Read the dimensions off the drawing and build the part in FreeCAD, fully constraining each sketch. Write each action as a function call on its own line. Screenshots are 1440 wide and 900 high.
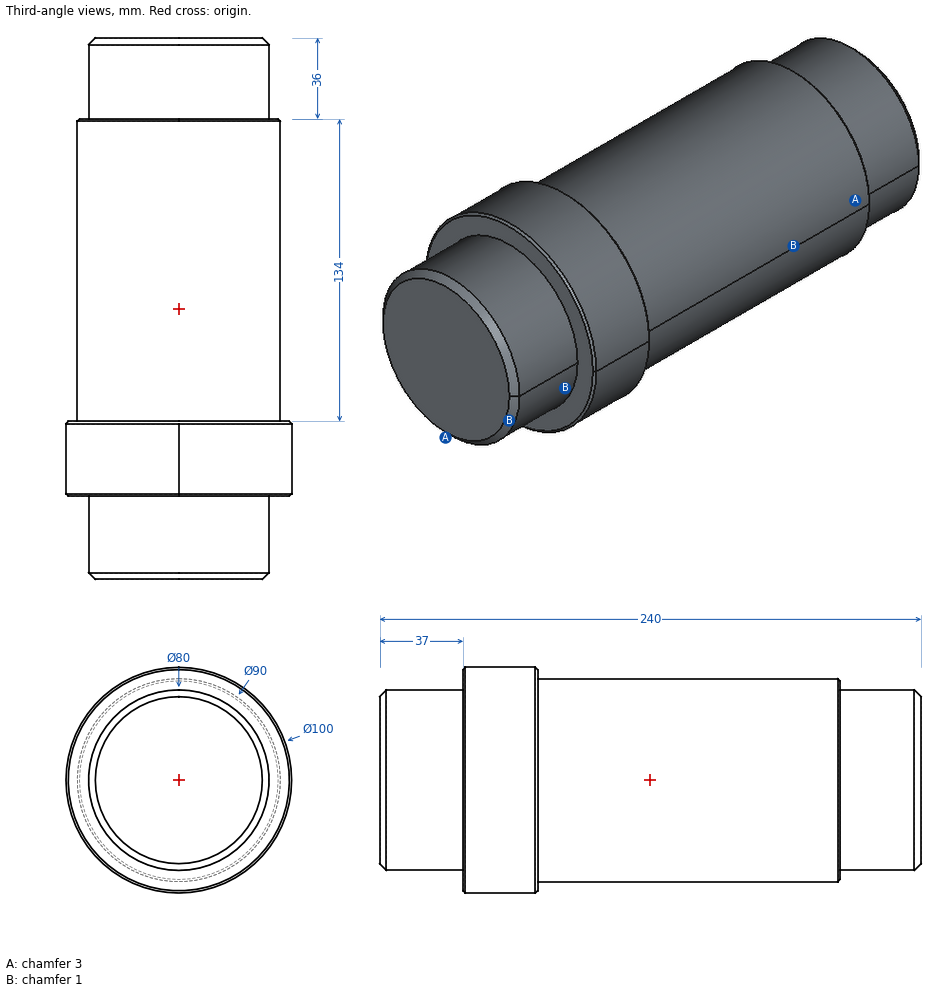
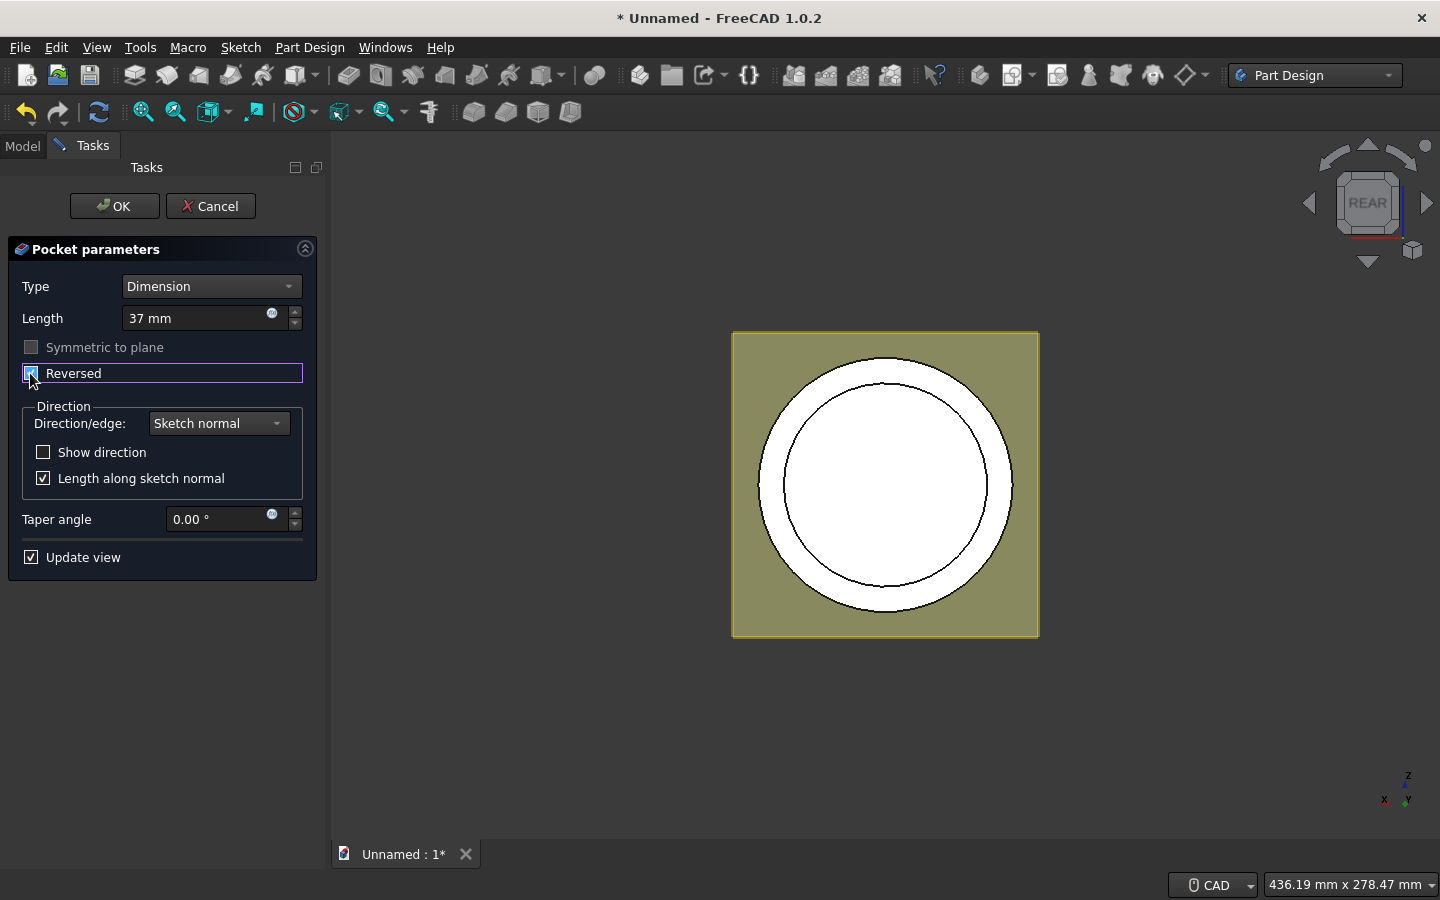
click(115, 206)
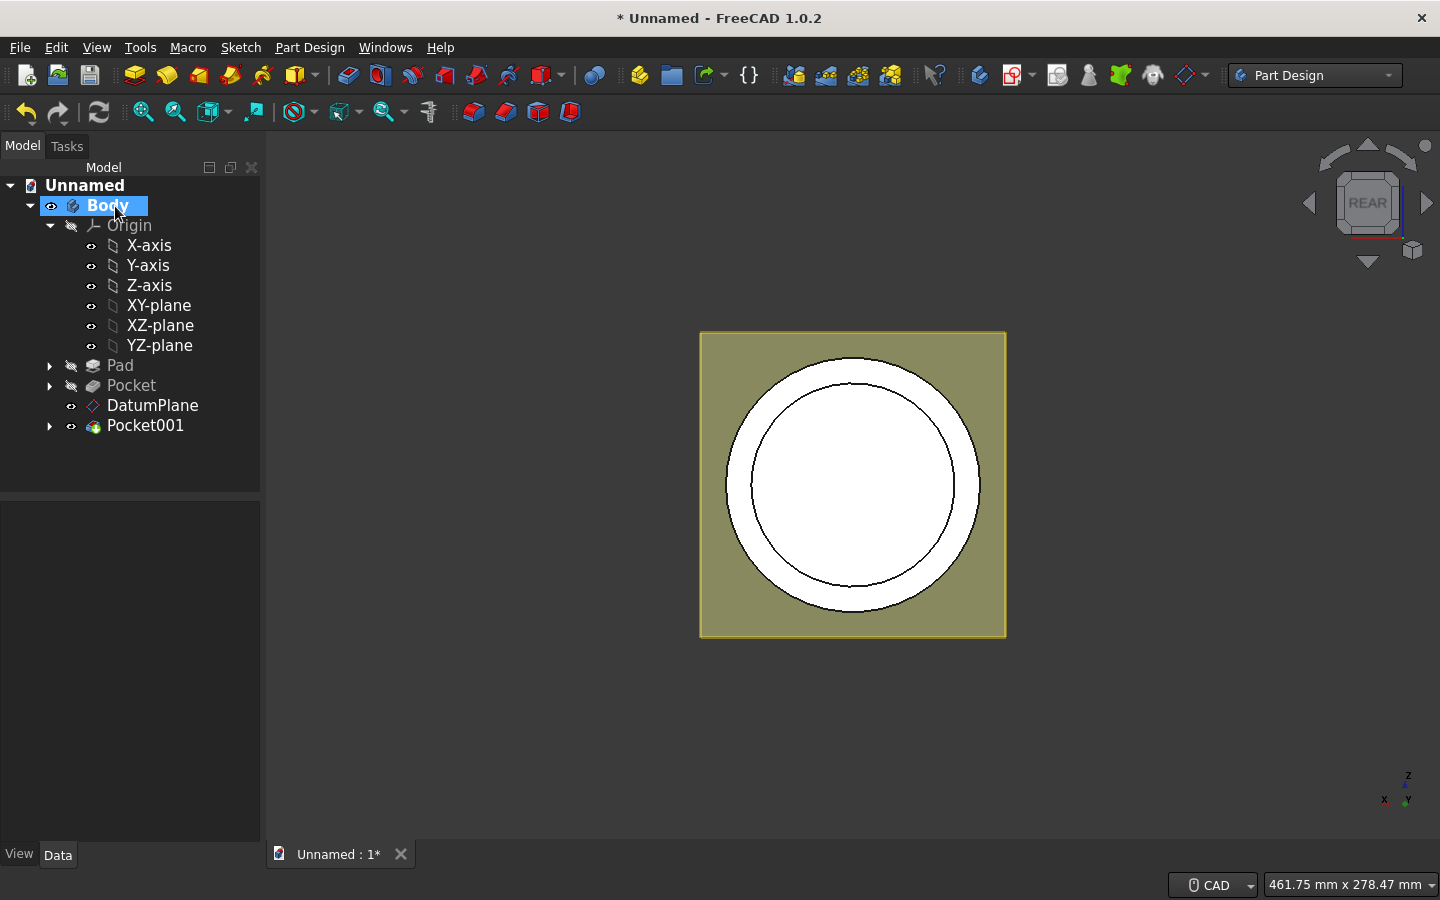
click(116, 406)
key(space)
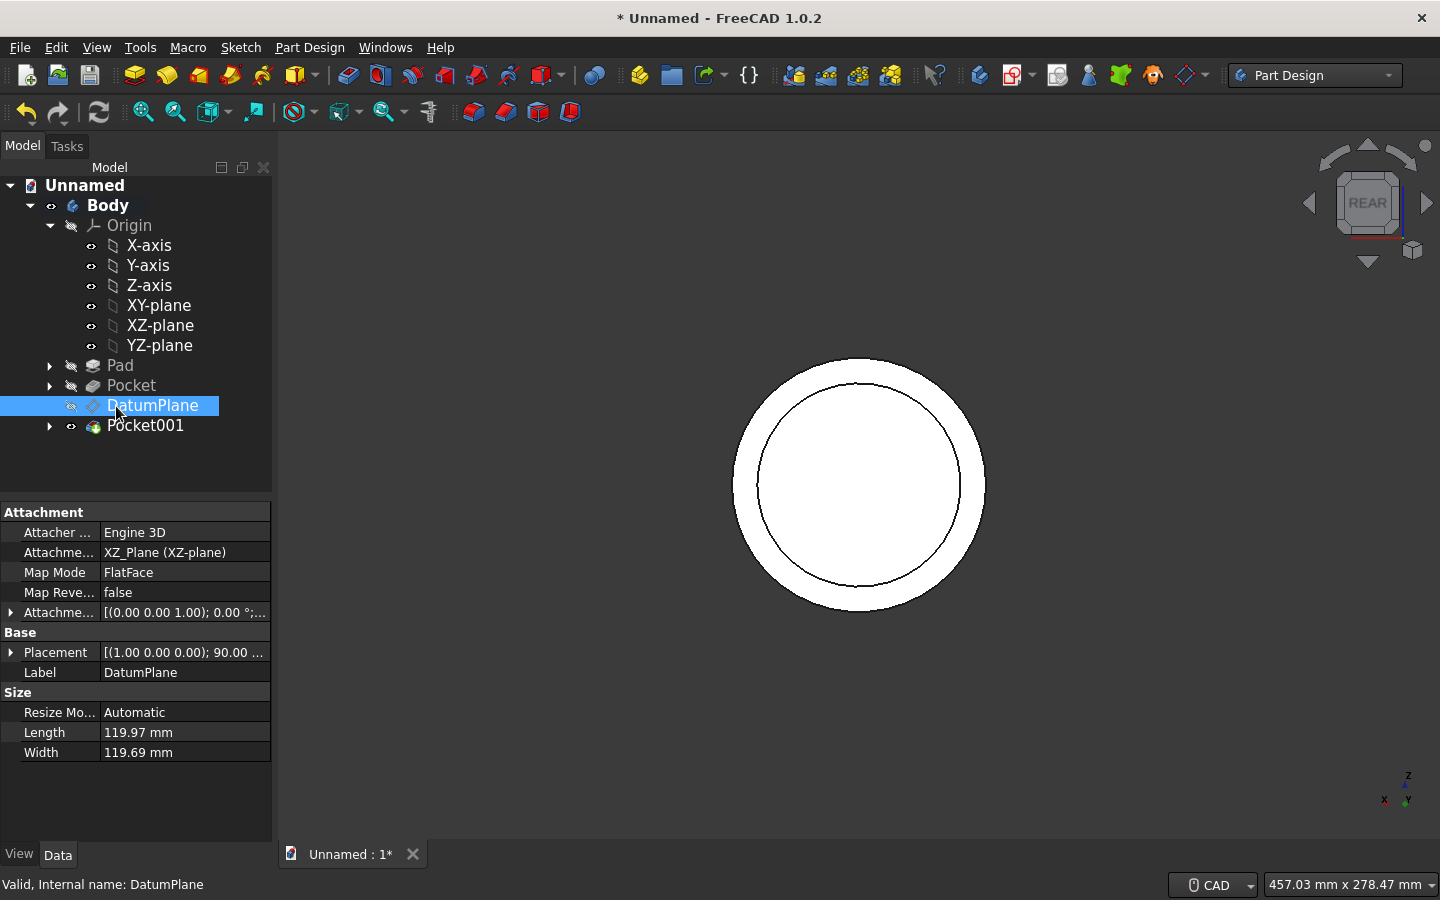
click(144, 112)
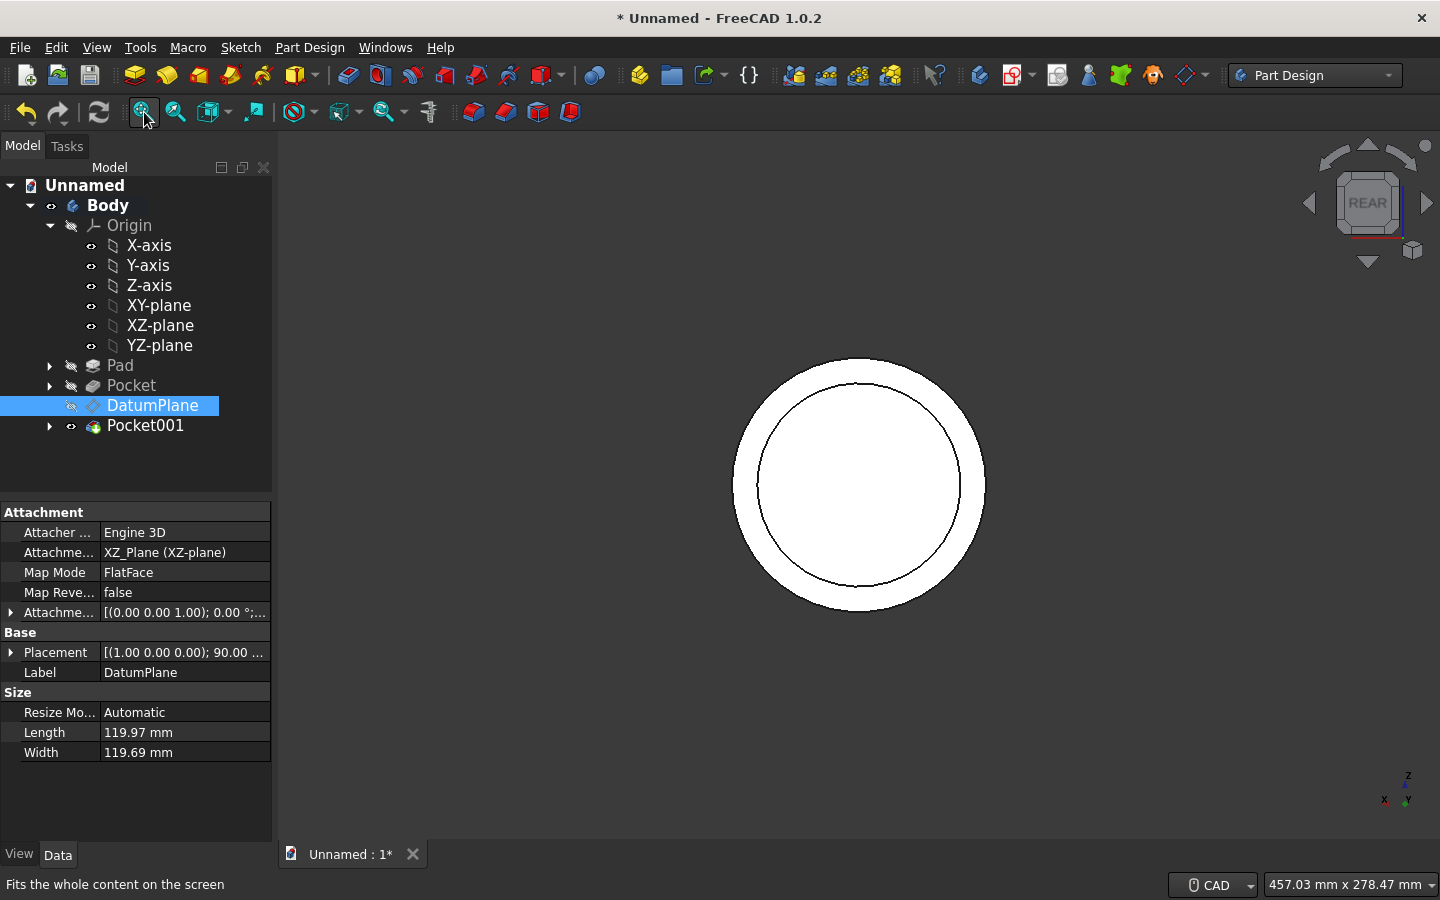
click(823, 593)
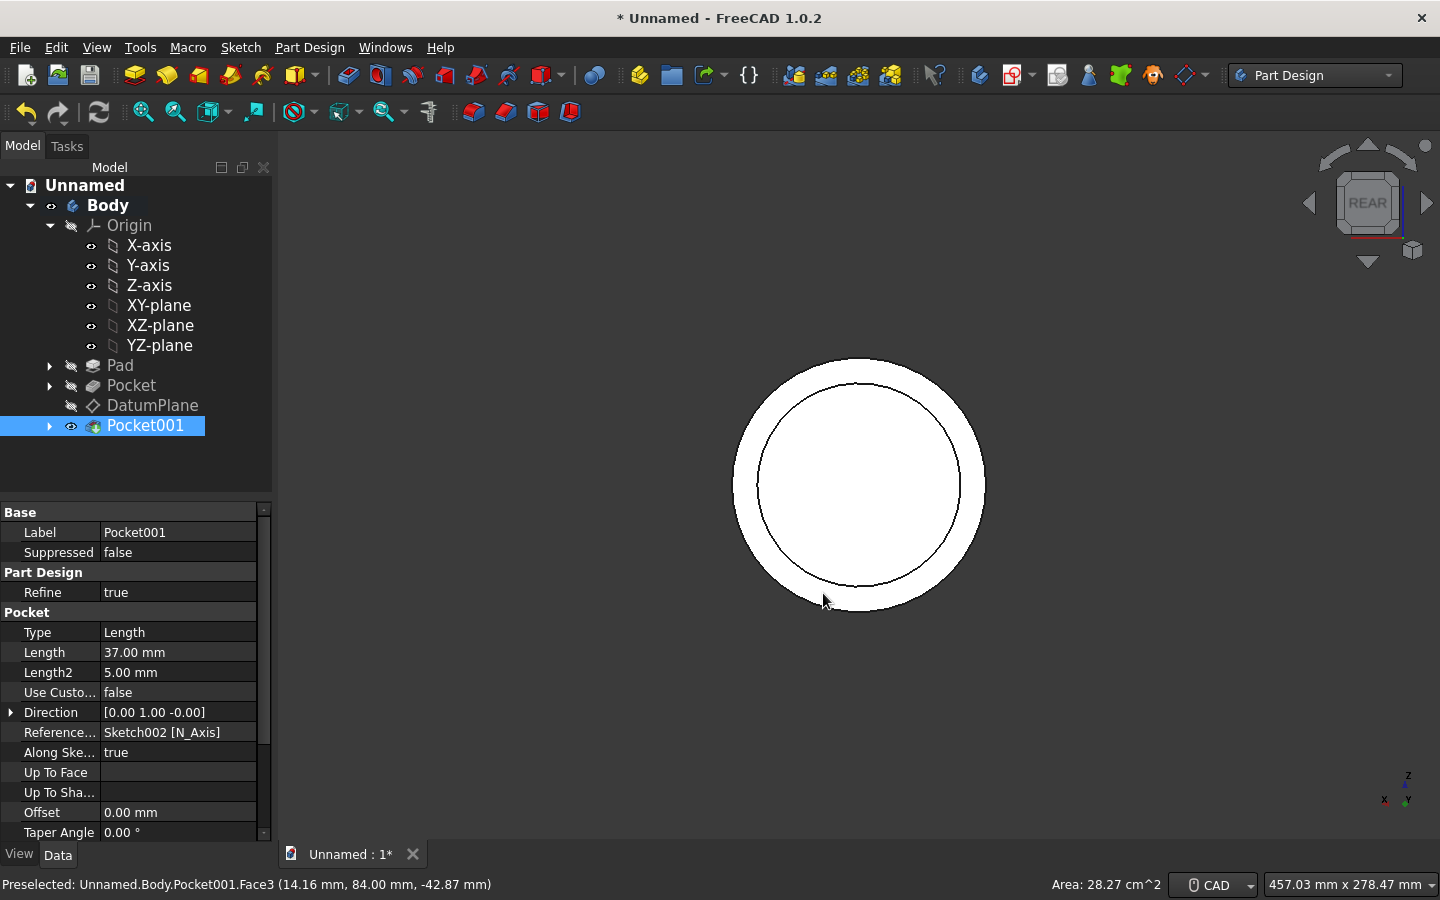
click(1012, 76)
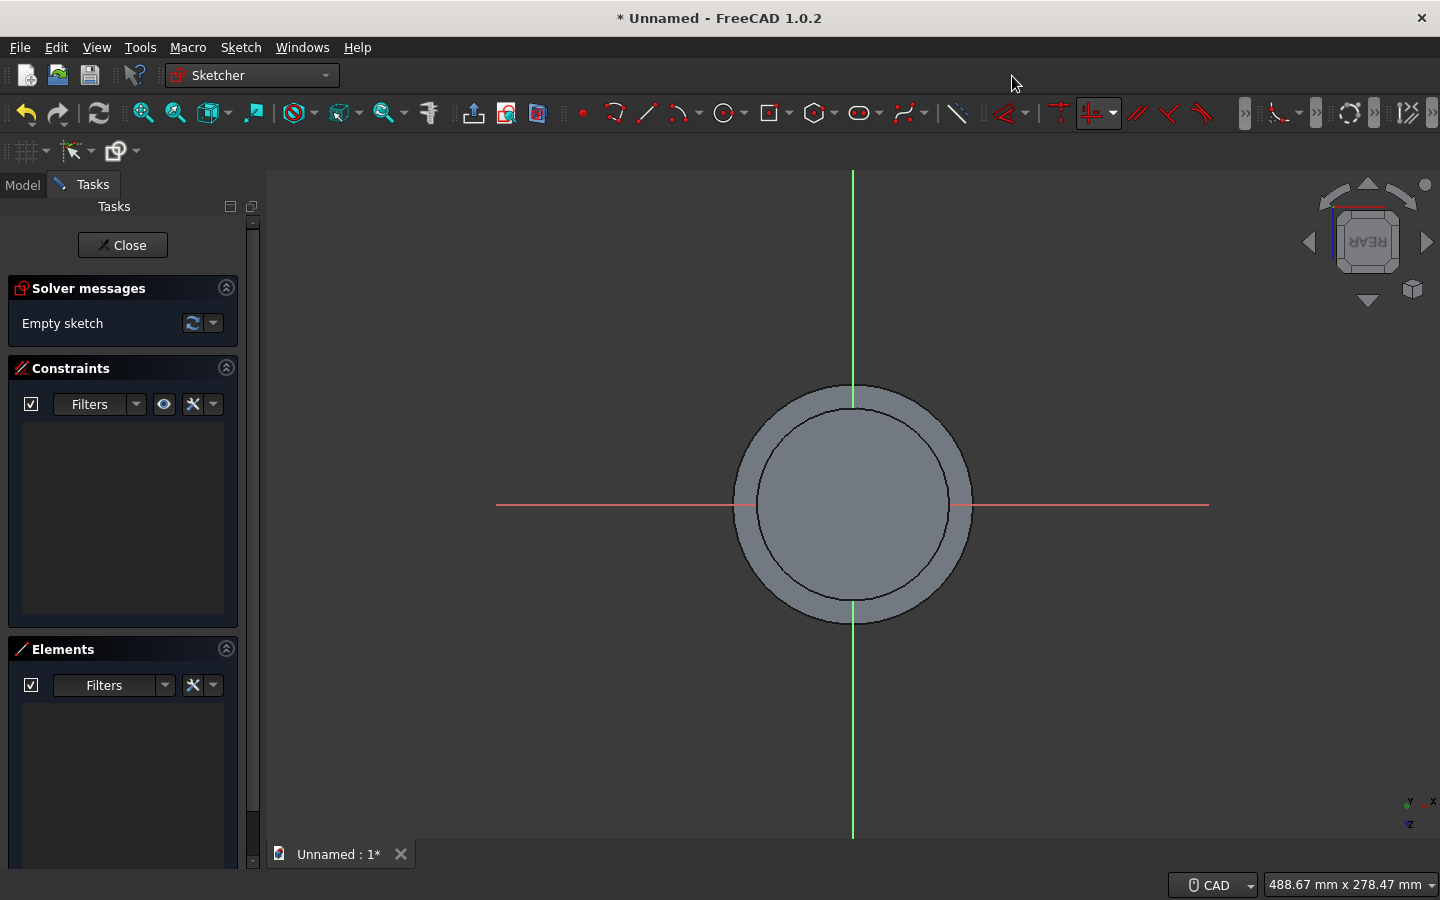
click(538, 114)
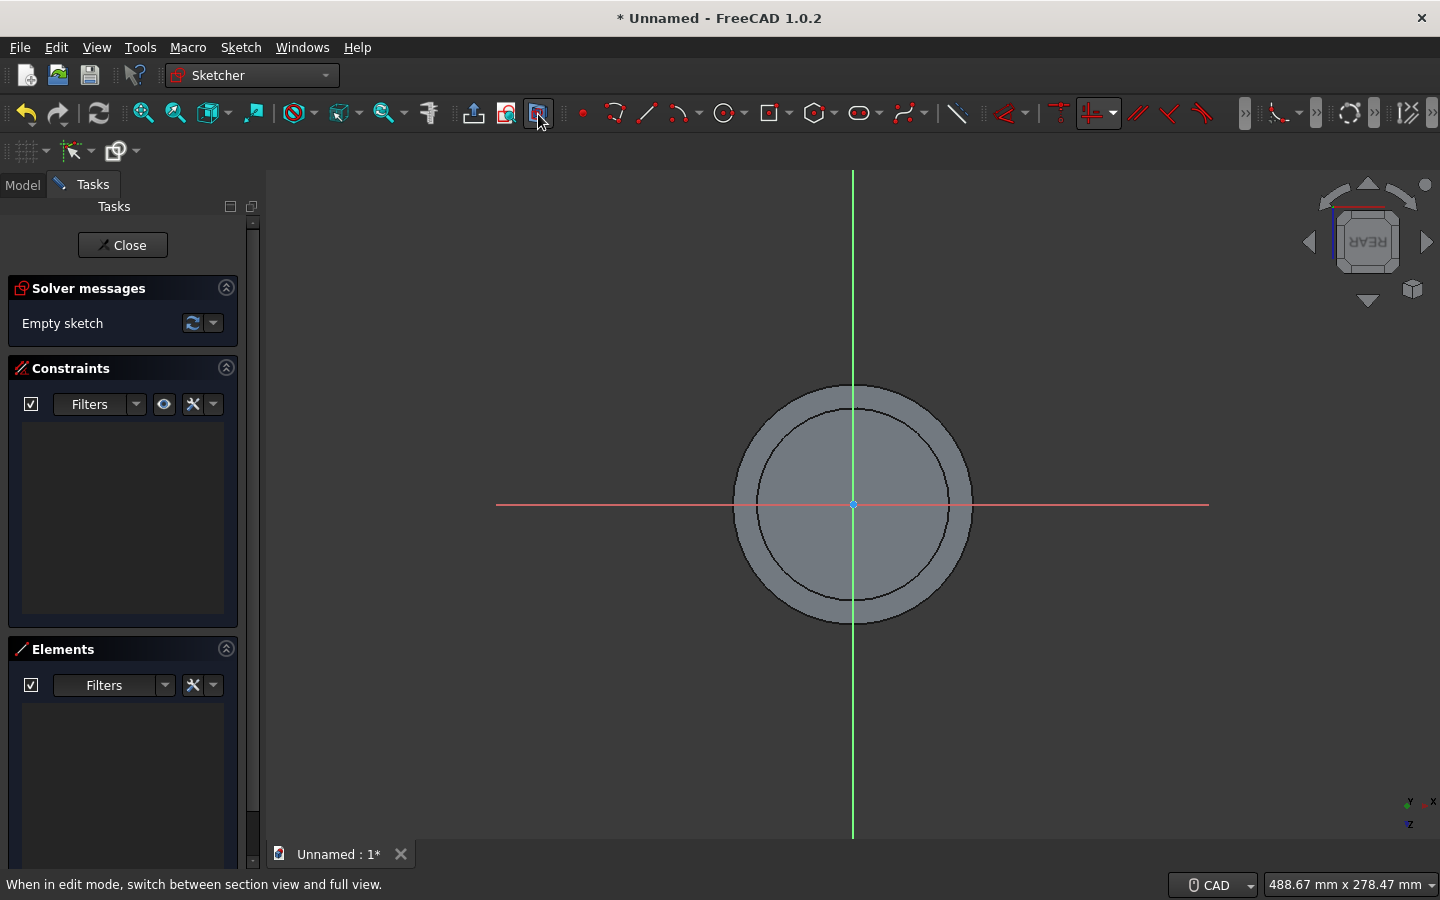
scroll(936, 505, up, 3)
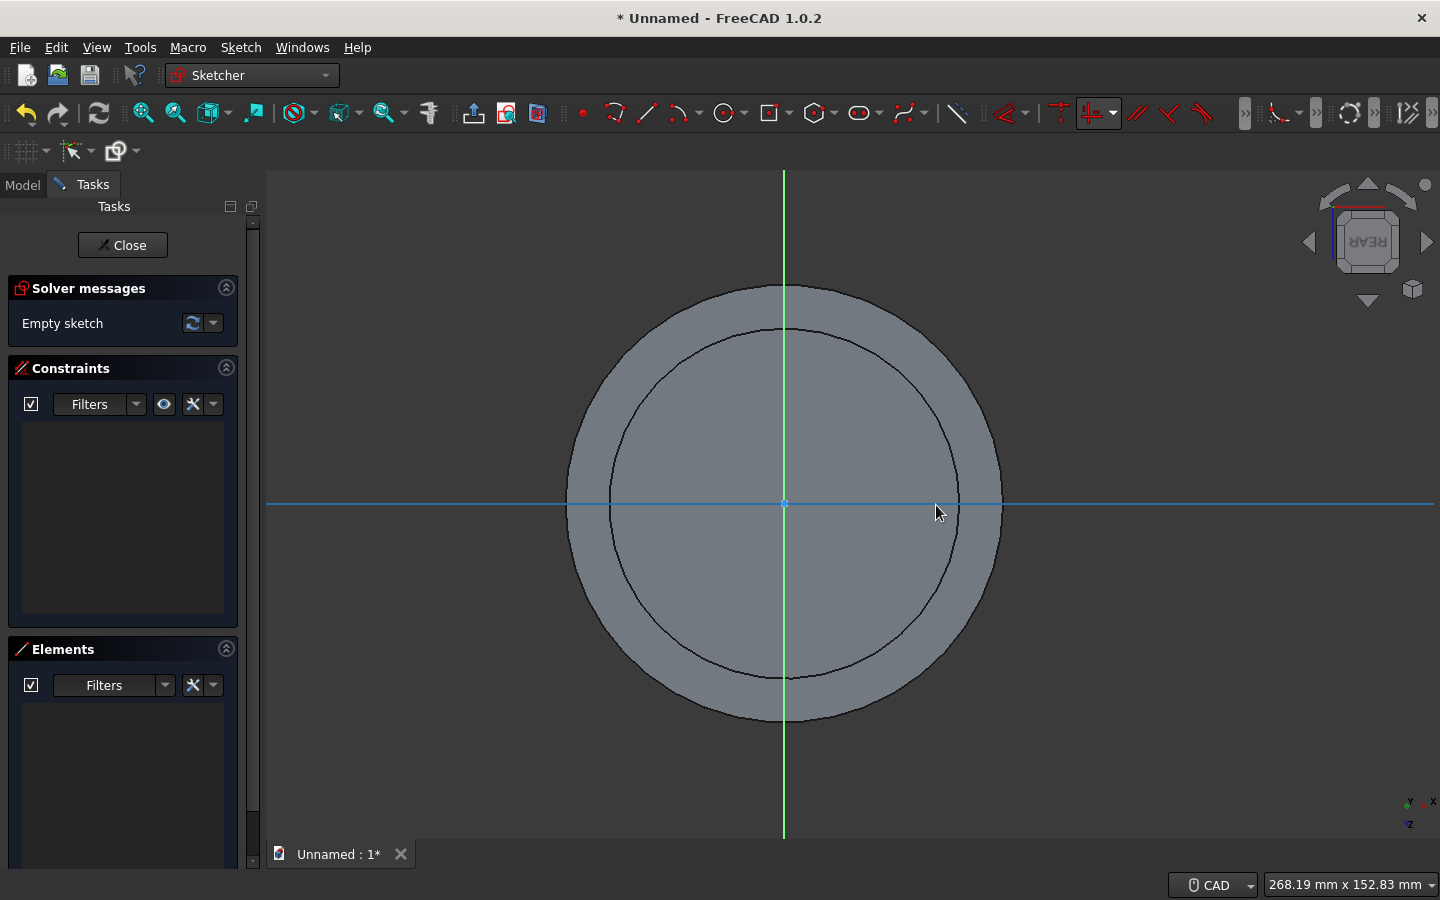
click(724, 114)